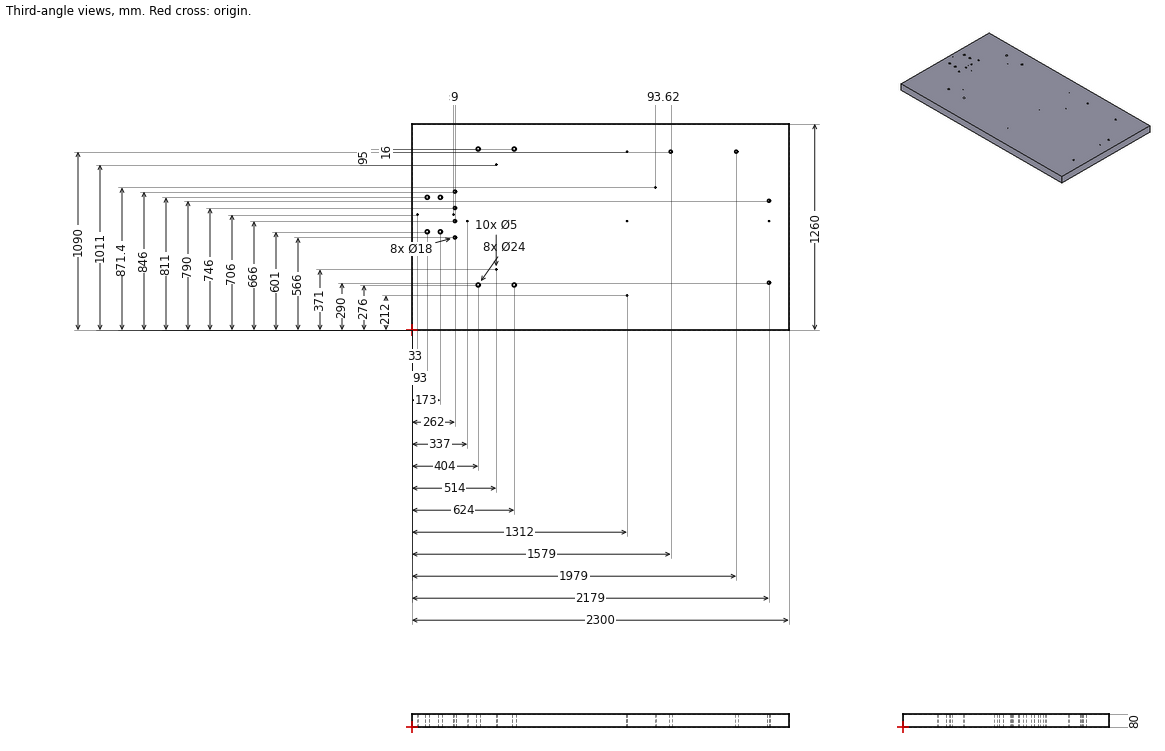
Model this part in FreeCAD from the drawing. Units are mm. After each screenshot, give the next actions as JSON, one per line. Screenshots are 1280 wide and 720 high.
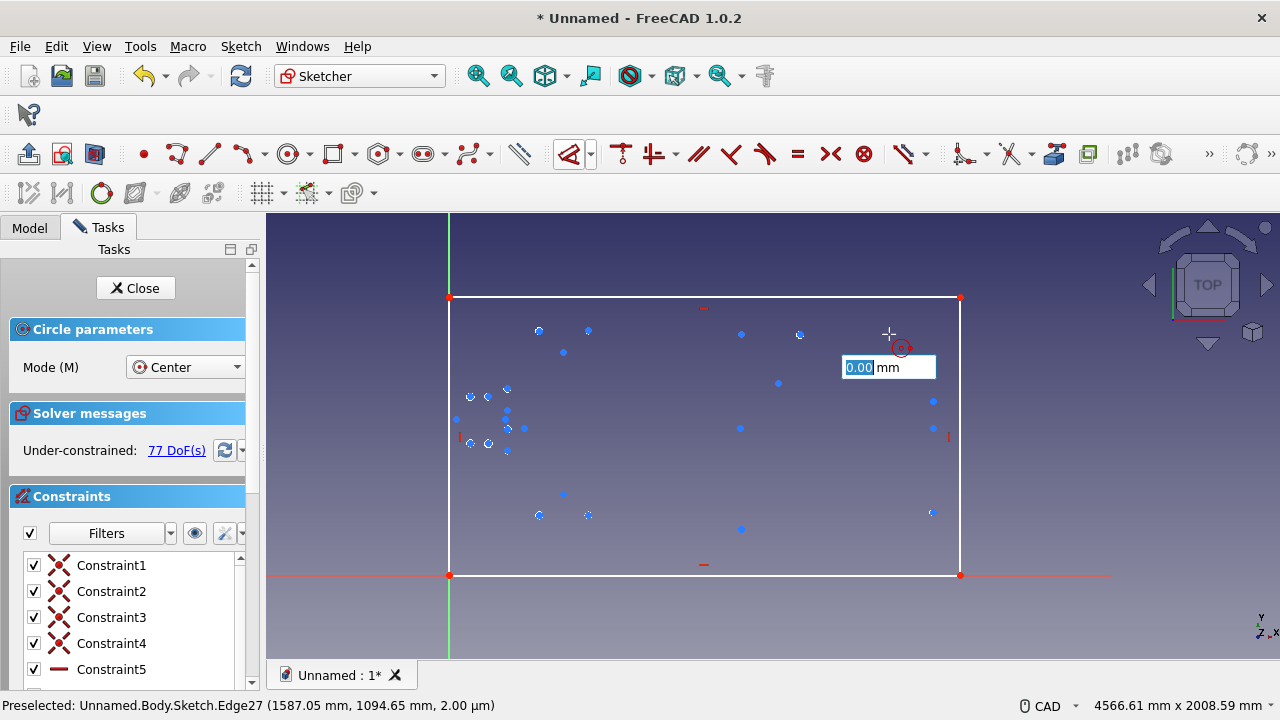
{"action": "scroll", "coordinate": [890, 332], "scroll_direction": "up", "scroll_amount": 11}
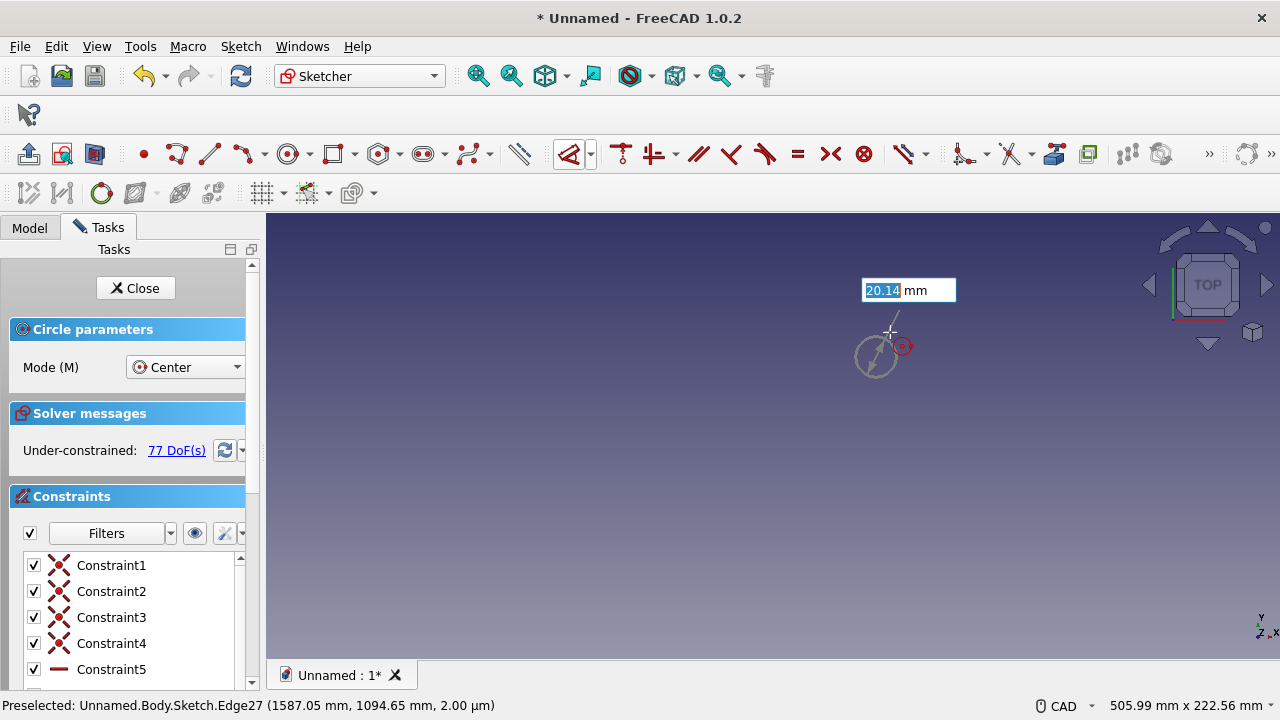
{"action": "left_click", "coordinate": [888, 333]}
{"action": "key", "text": "Escape"}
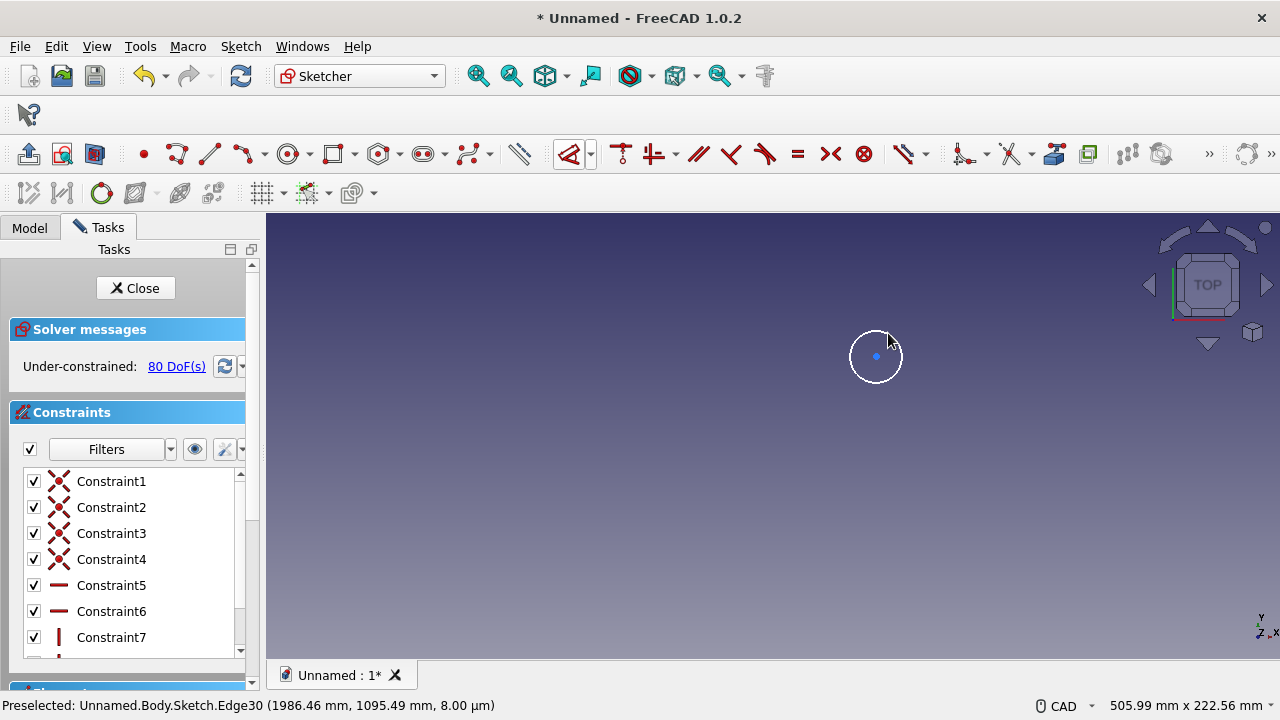
{"action": "scroll", "coordinate": [890, 332], "scroll_direction": "down", "scroll_amount": 11}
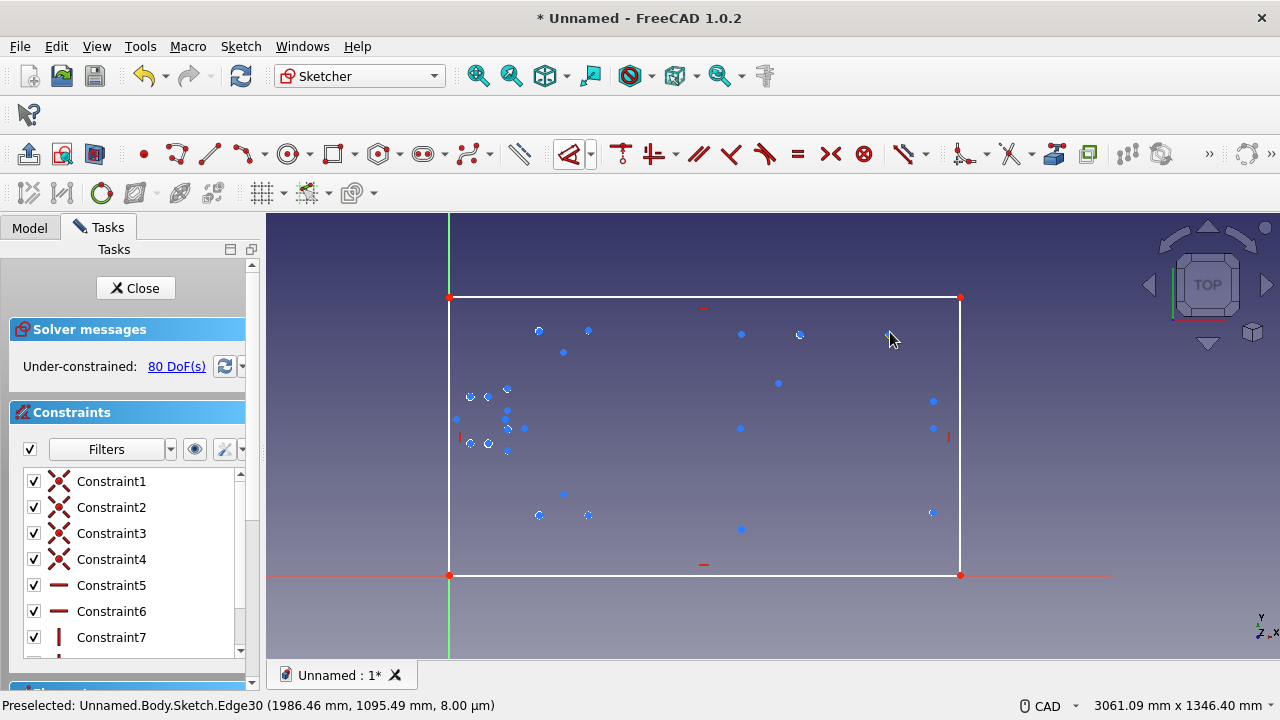
{"action": "scroll", "coordinate": [542, 513], "scroll_direction": "up", "scroll_amount": 8}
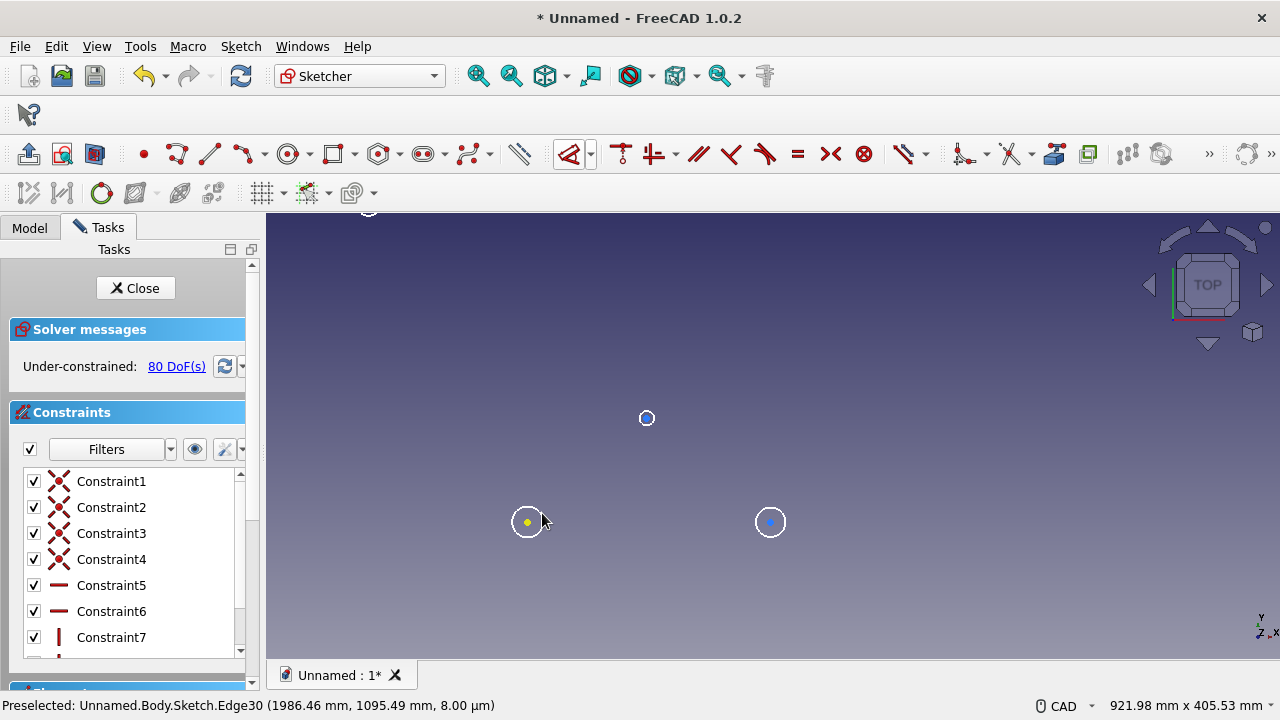
{"action": "left_click", "coordinate": [539, 511]}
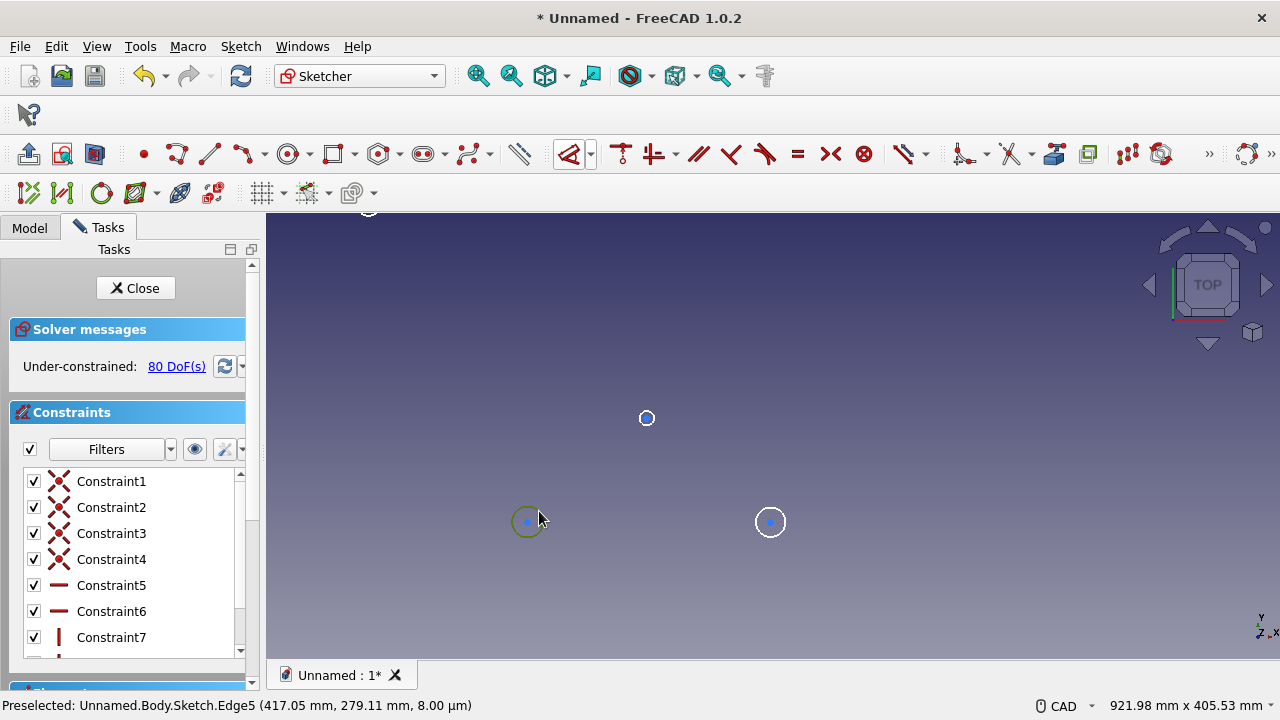
{"action": "left_click", "coordinate": [781, 512]}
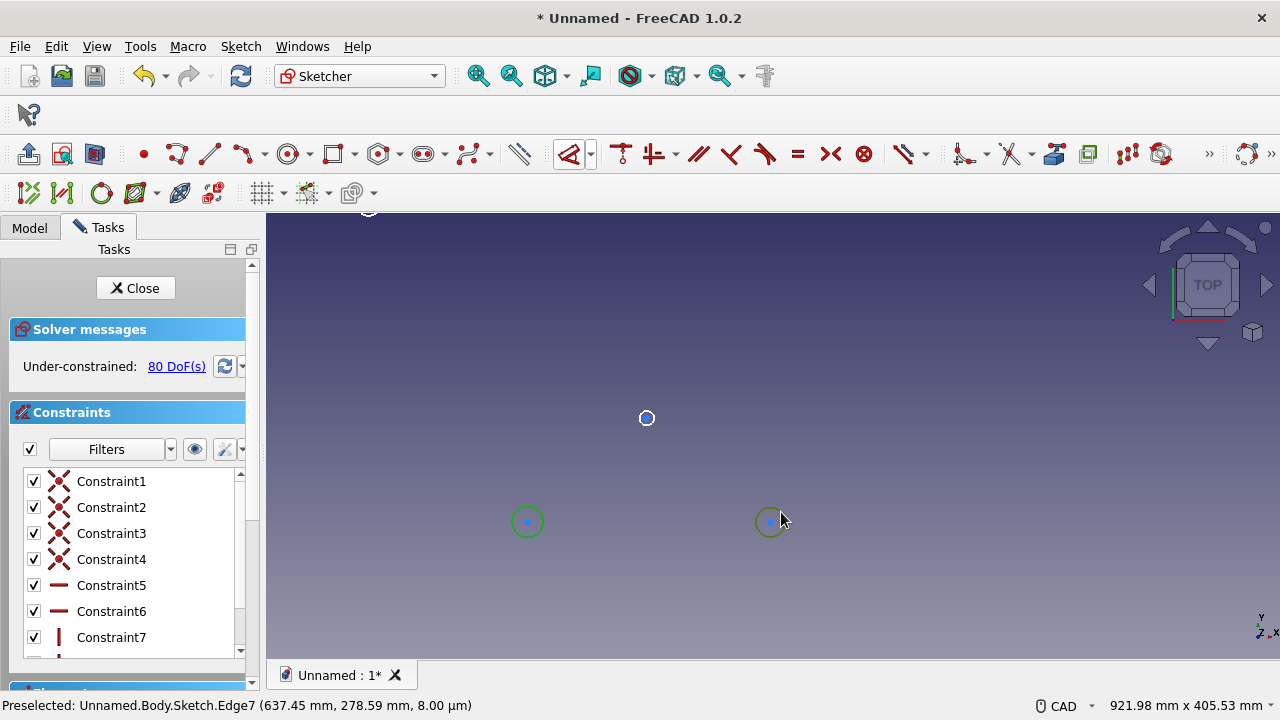
{"action": "scroll", "coordinate": [542, 514], "scroll_direction": "down", "scroll_amount": 8}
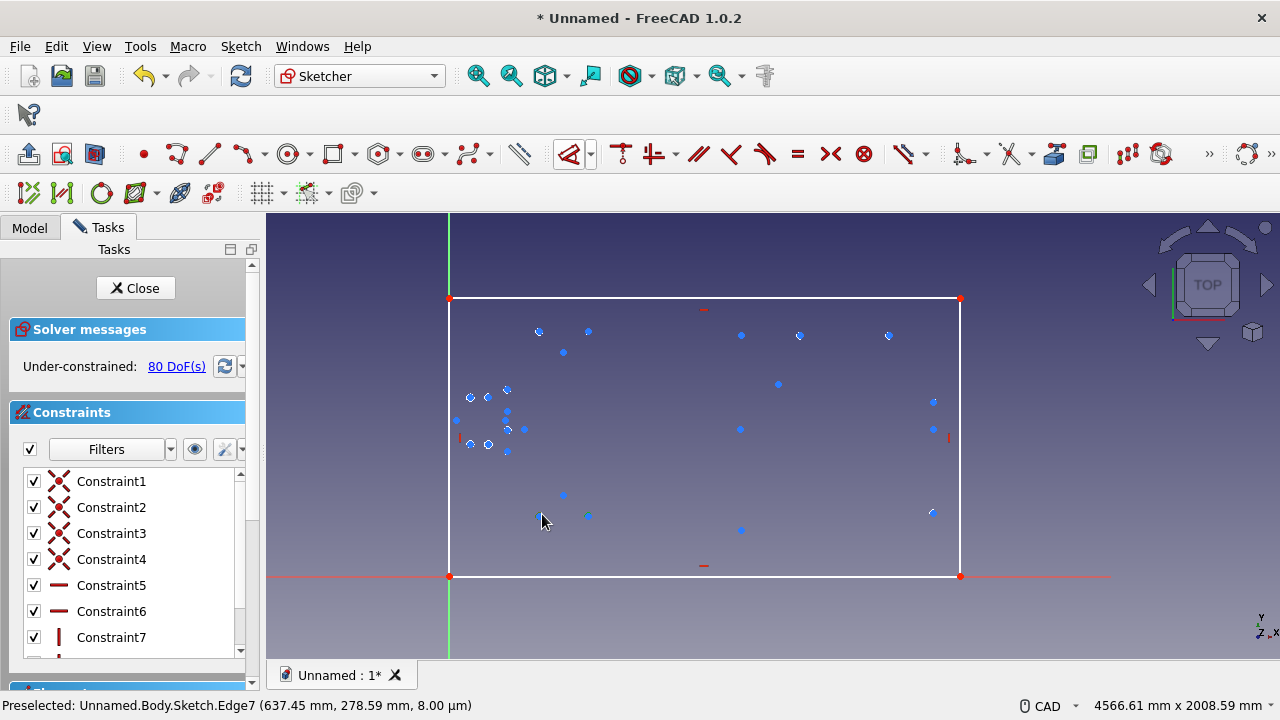
{"action": "scroll", "coordinate": [473, 442], "scroll_direction": "up", "scroll_amount": 8}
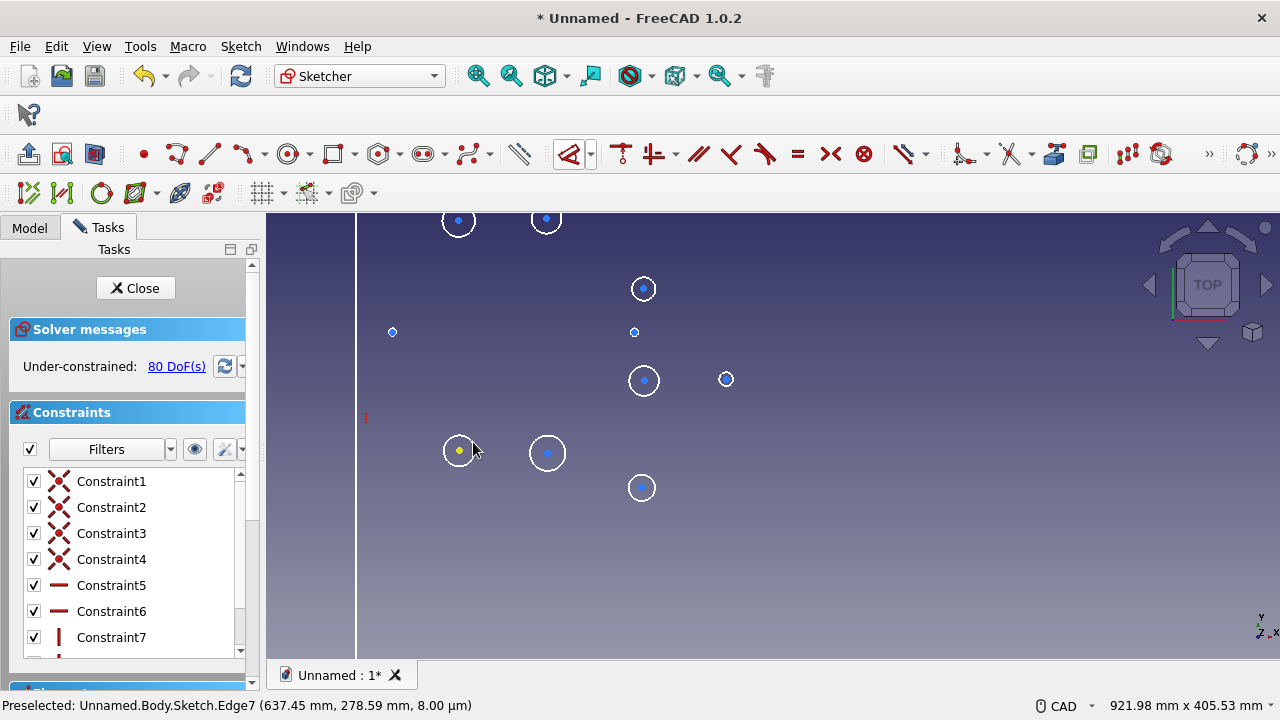
{"action": "left_click", "coordinate": [470, 440]}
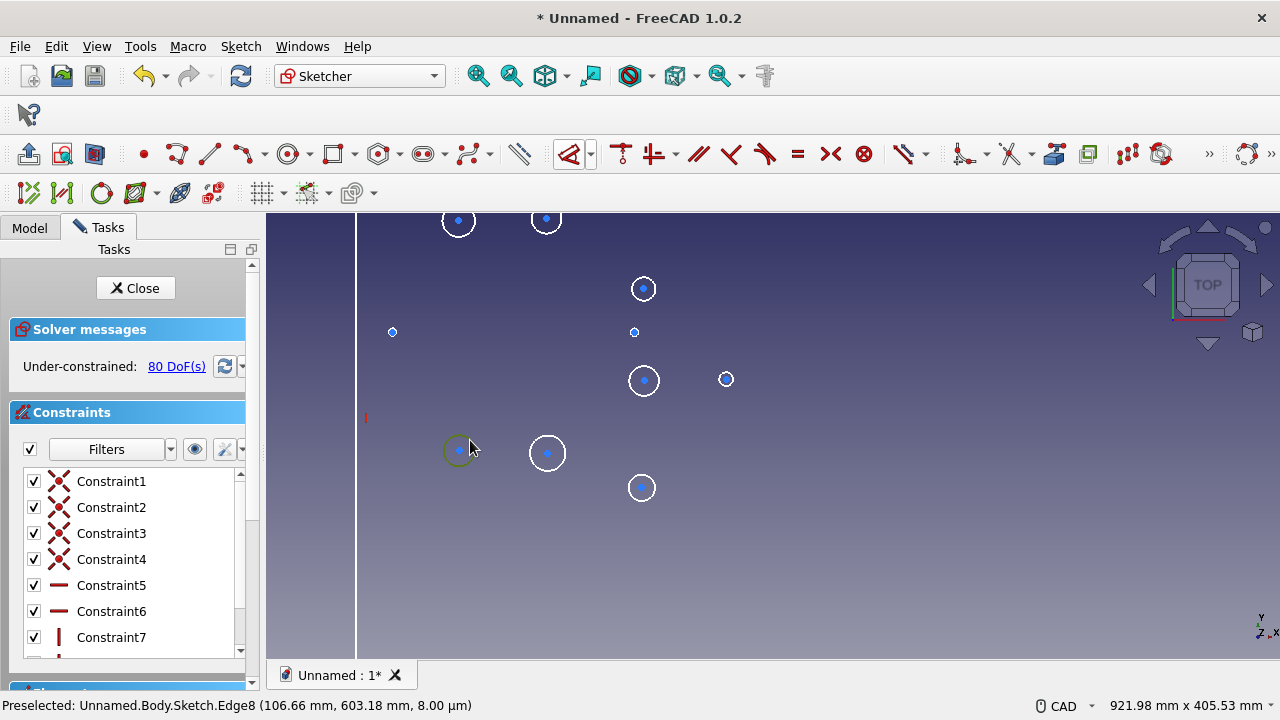
{"action": "left_click", "coordinate": [560, 441]}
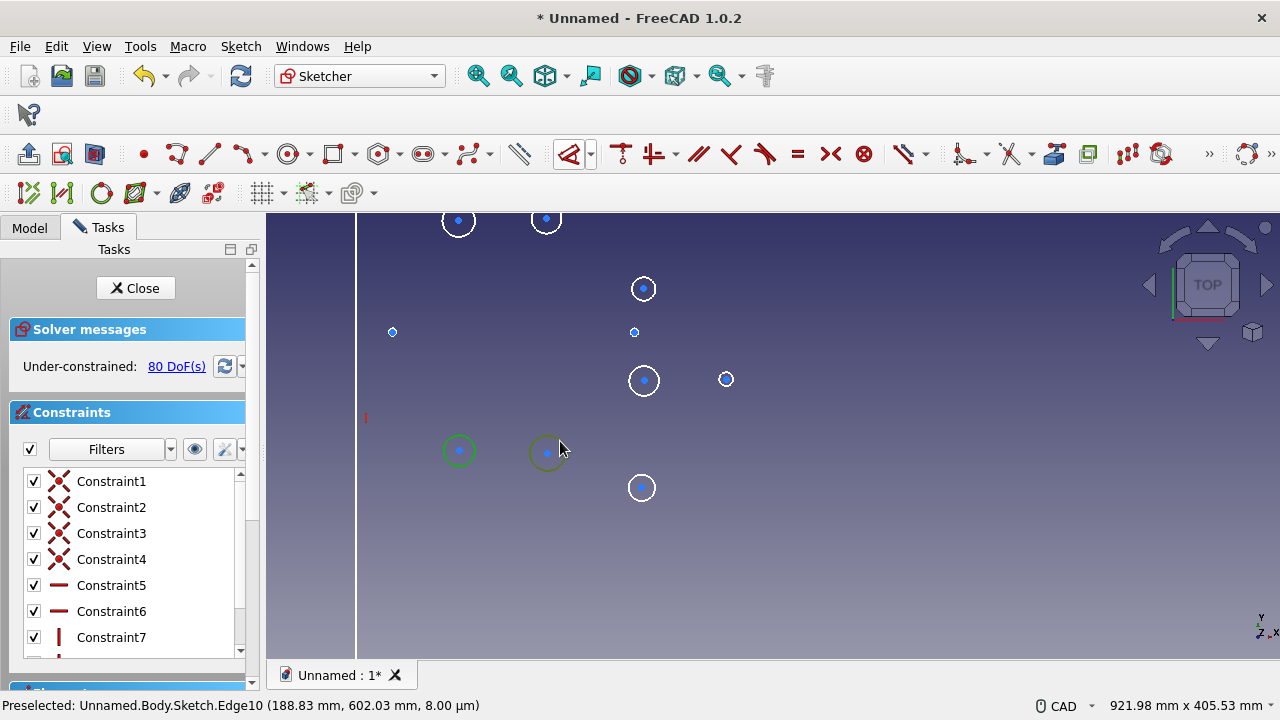
{"action": "scroll", "coordinate": [473, 442], "scroll_direction": "down", "scroll_amount": 8}